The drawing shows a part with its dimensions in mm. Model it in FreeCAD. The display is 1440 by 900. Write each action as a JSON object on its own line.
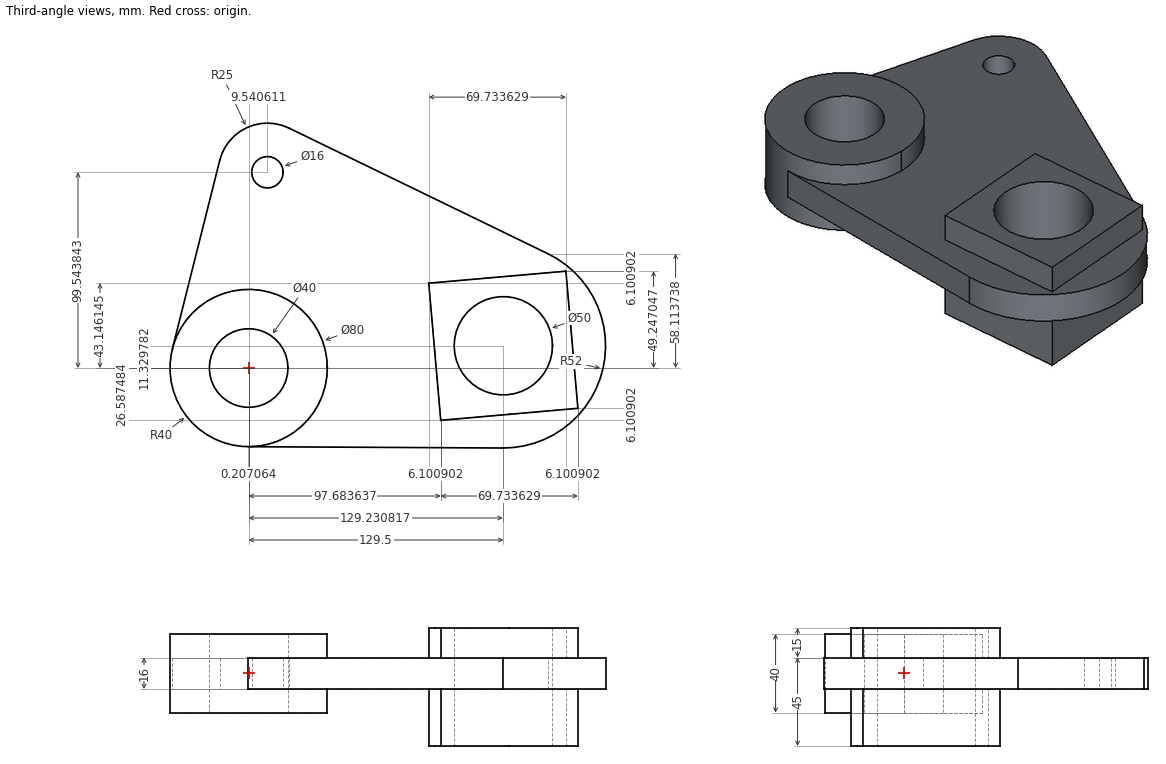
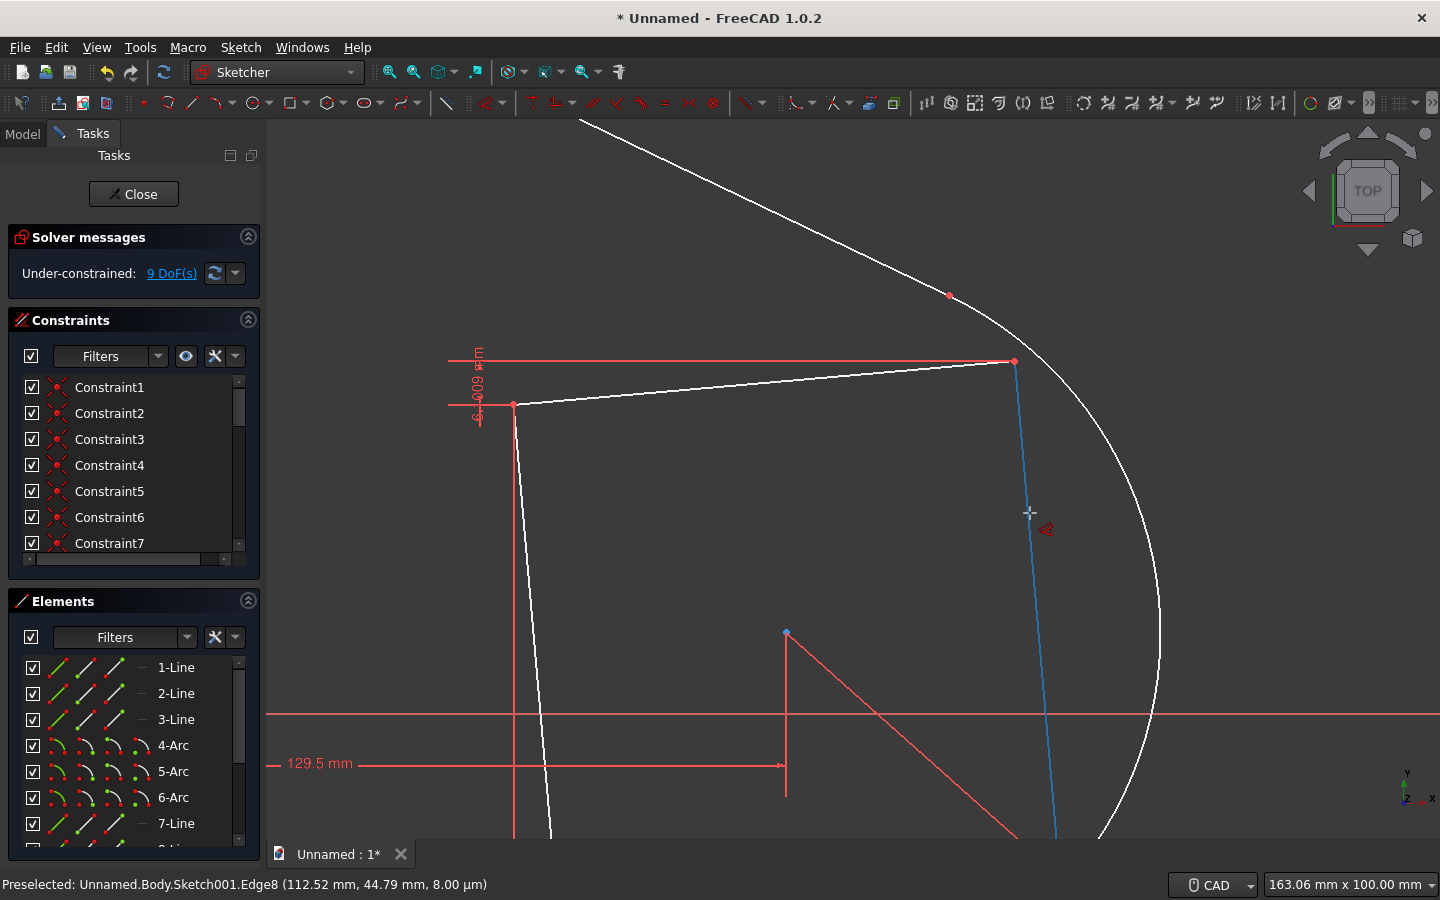
{"action": "left_click", "coordinate": [1028, 512]}
{"action": "left_click", "coordinate": [1037, 327]}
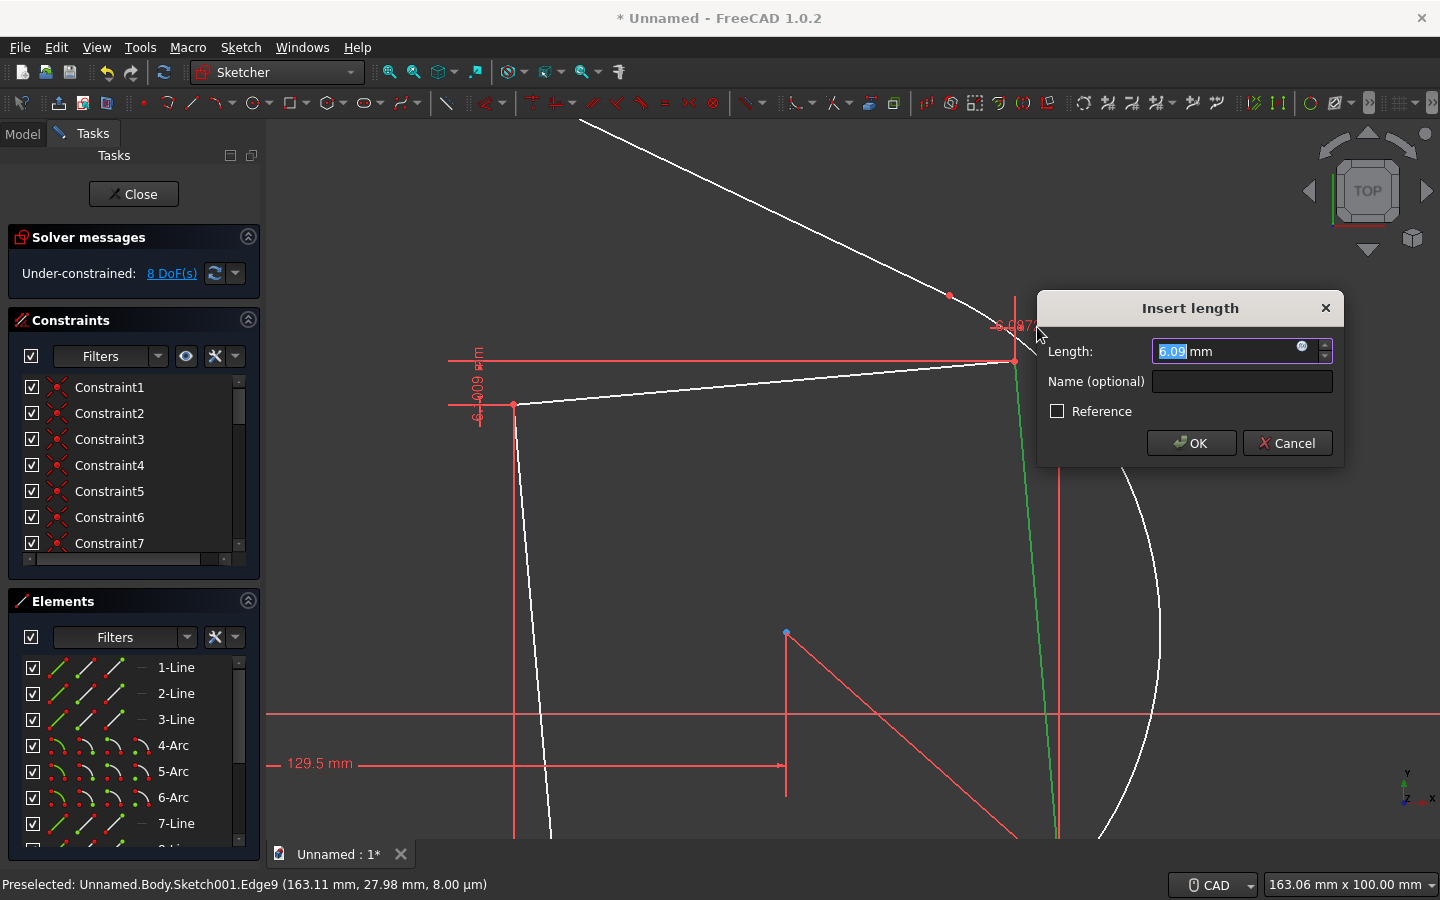
{"action": "type", "text": "6.100902"}
{"action": "key", "text": "Return"}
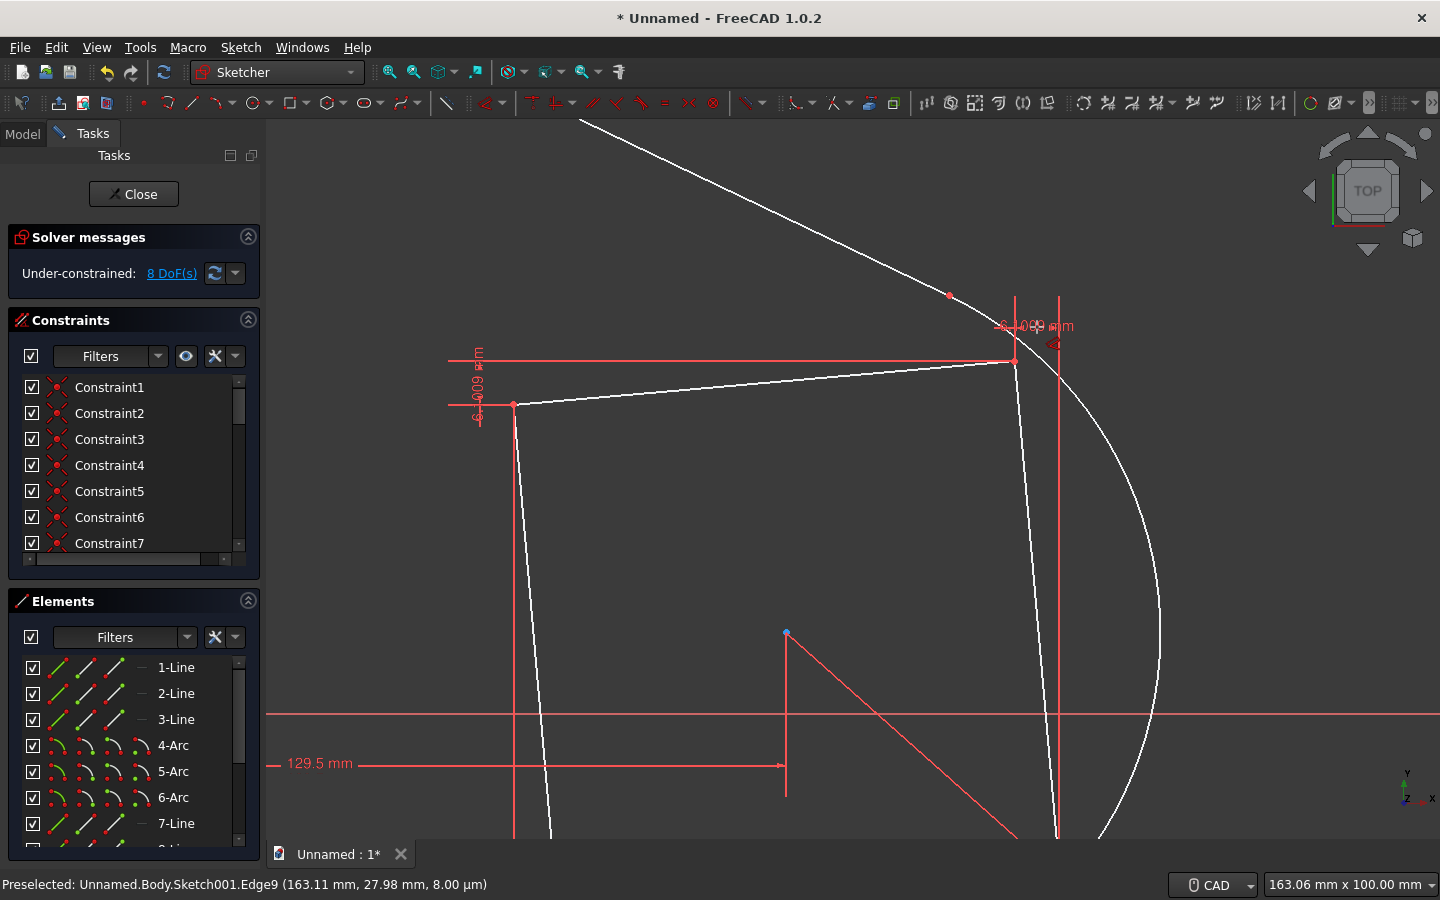
{"action": "scroll", "coordinate": [1030, 513], "scroll_direction": "down", "scroll_amount": 5}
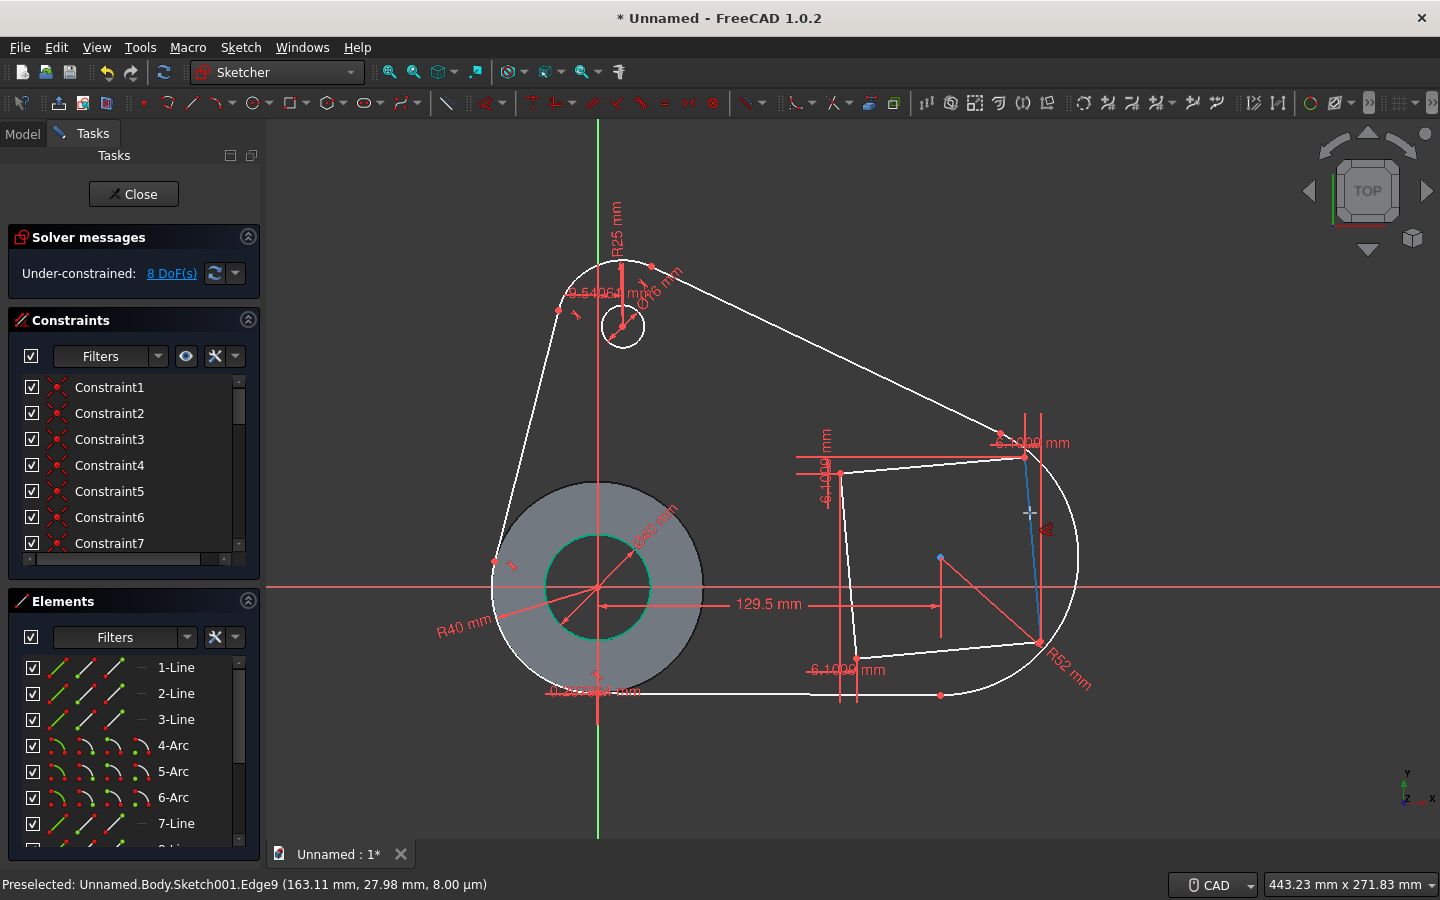
{"action": "scroll", "coordinate": [986, 647], "scroll_direction": "up", "scroll_amount": 5}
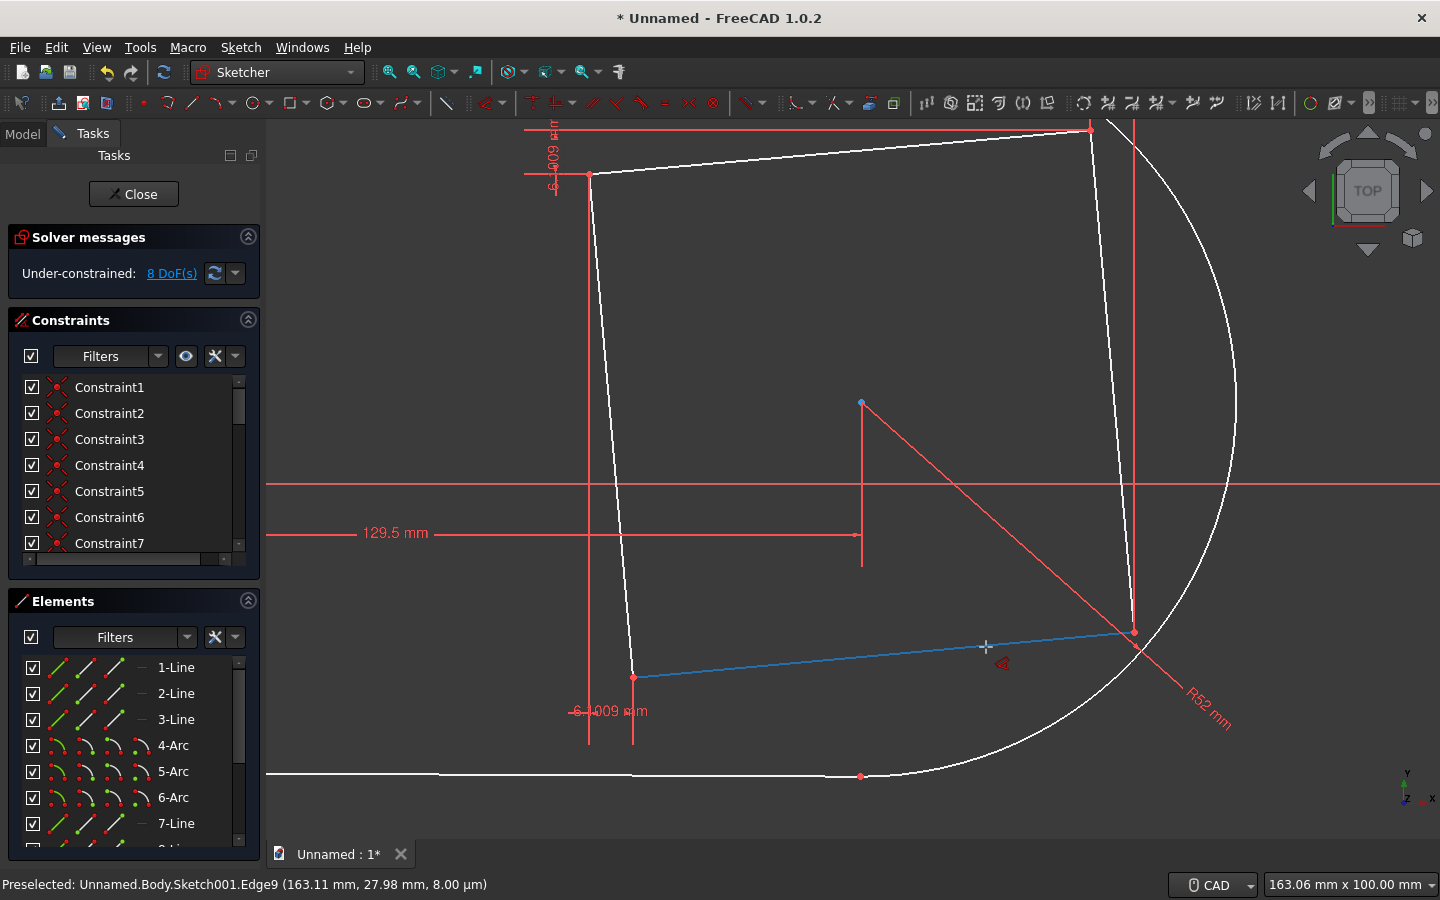
{"action": "left_click", "coordinate": [984, 646]}
{"action": "left_click", "coordinate": [1168, 655]}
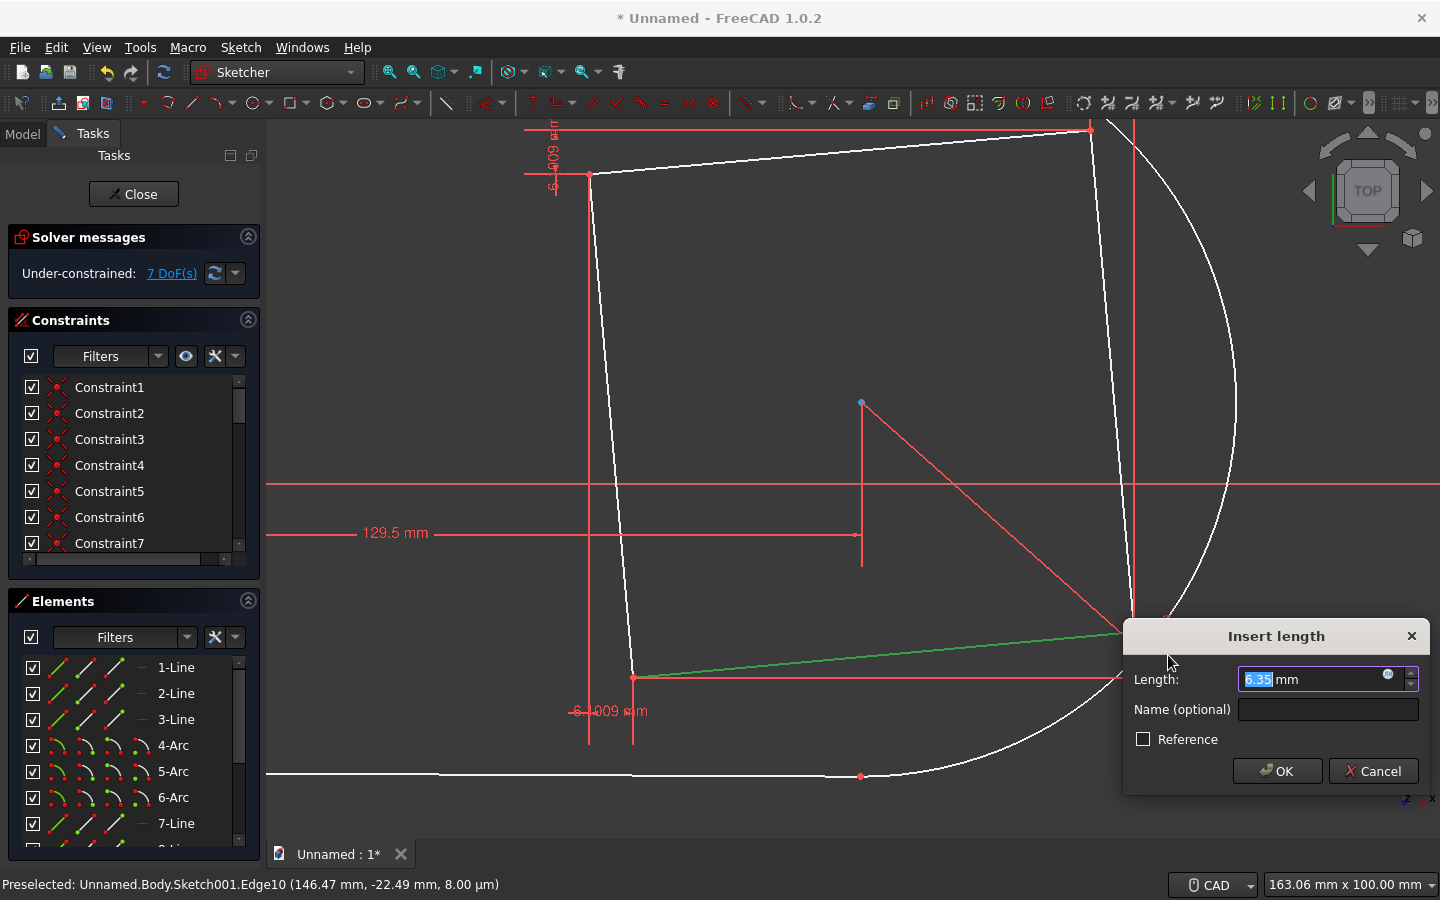
{"action": "type", "text": "6.100902"}
{"action": "key", "text": "Return"}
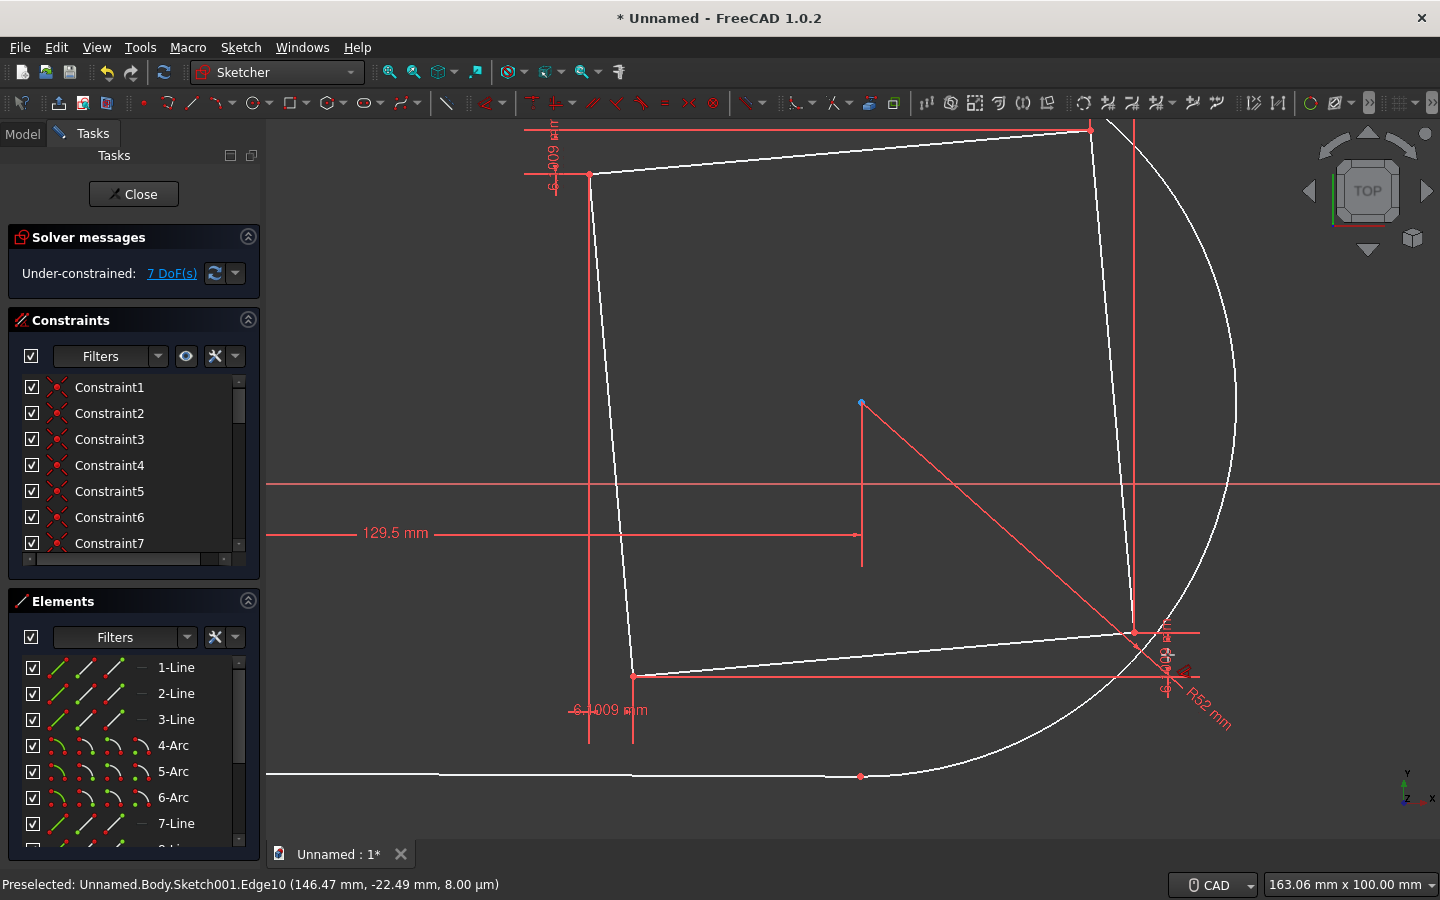
{"action": "scroll", "coordinate": [986, 647], "scroll_direction": "down", "scroll_amount": 5}